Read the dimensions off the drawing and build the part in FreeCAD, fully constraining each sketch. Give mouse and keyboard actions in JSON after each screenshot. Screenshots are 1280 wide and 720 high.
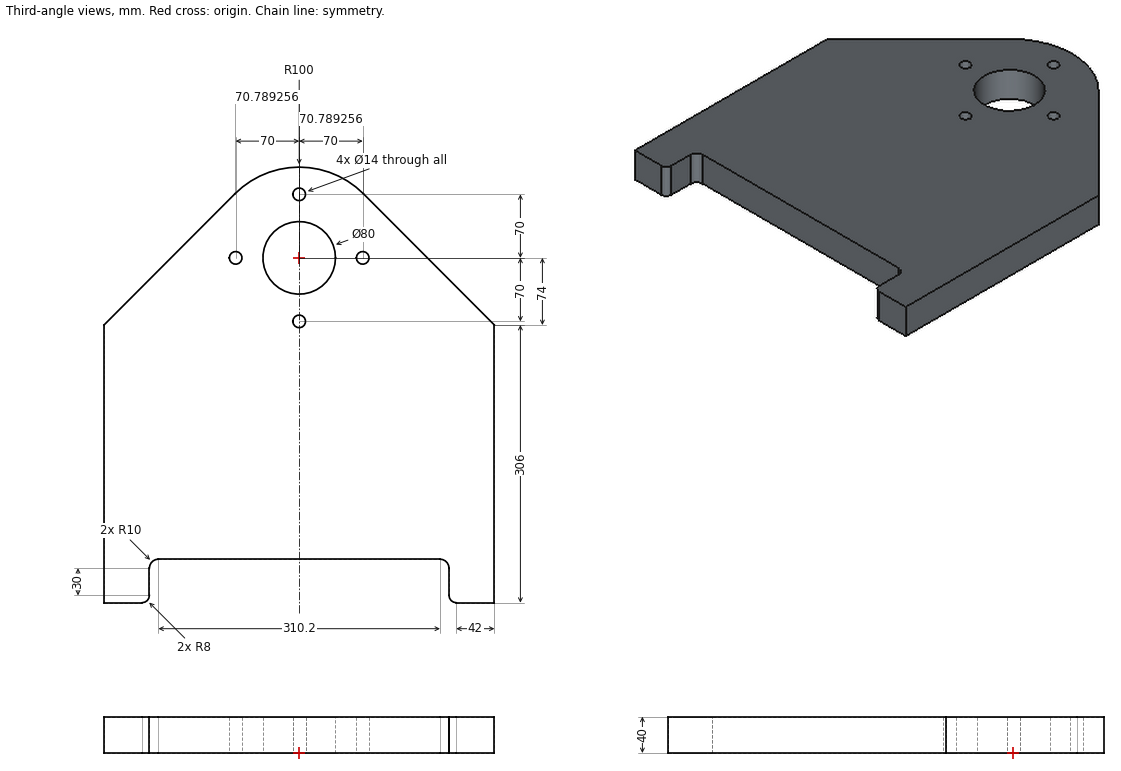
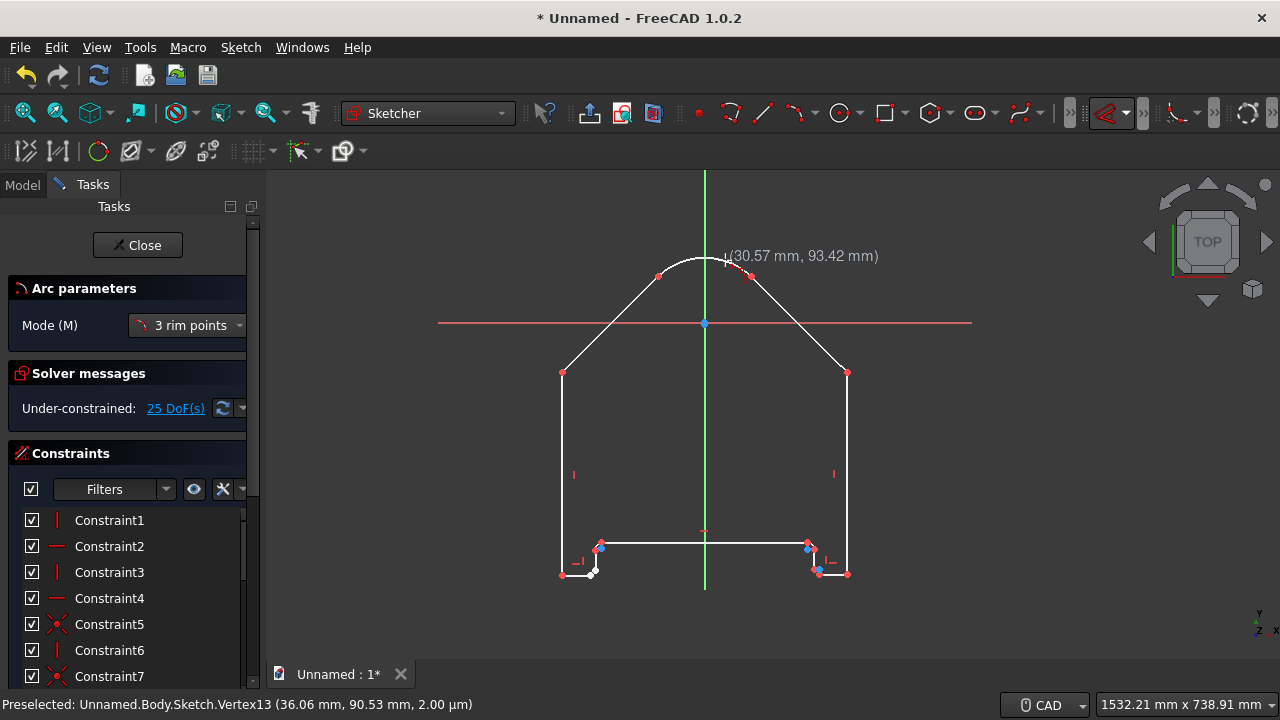
{"action": "scroll", "coordinate": [590, 574], "scroll_direction": "up", "scroll_amount": 4}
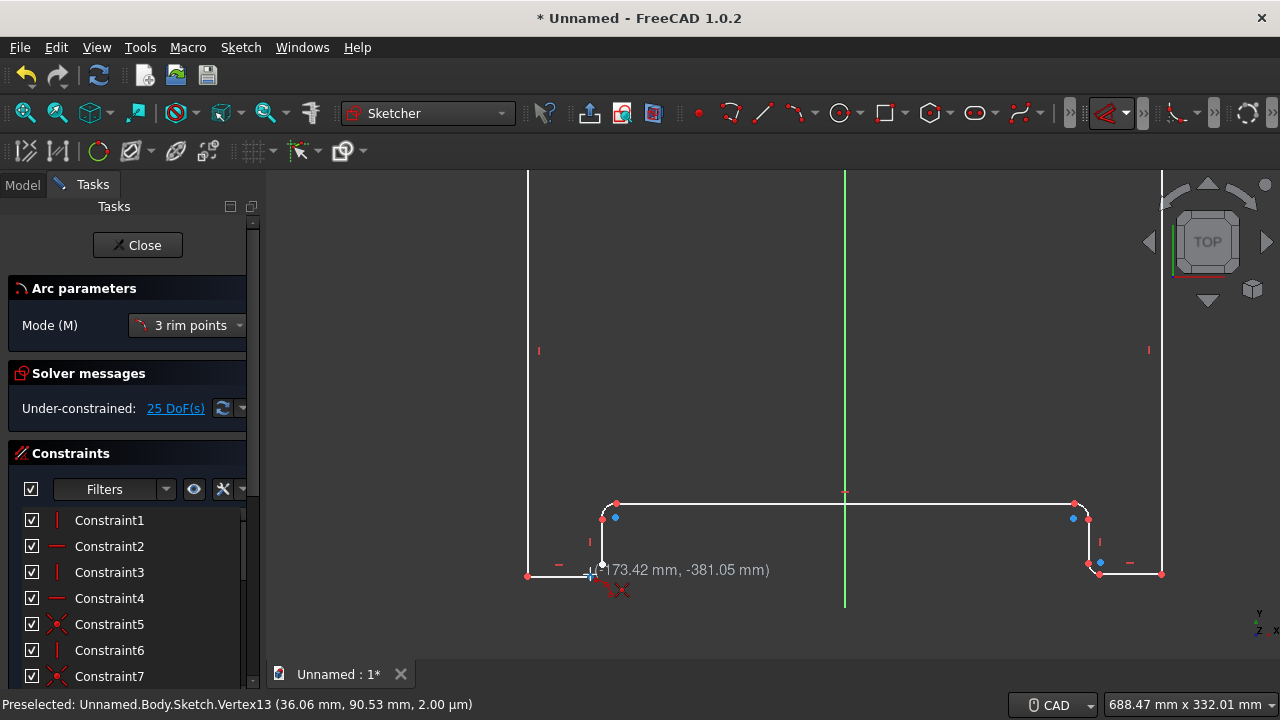
{"action": "left_click", "coordinate": [590, 577]}
{"action": "left_click", "coordinate": [602, 564]}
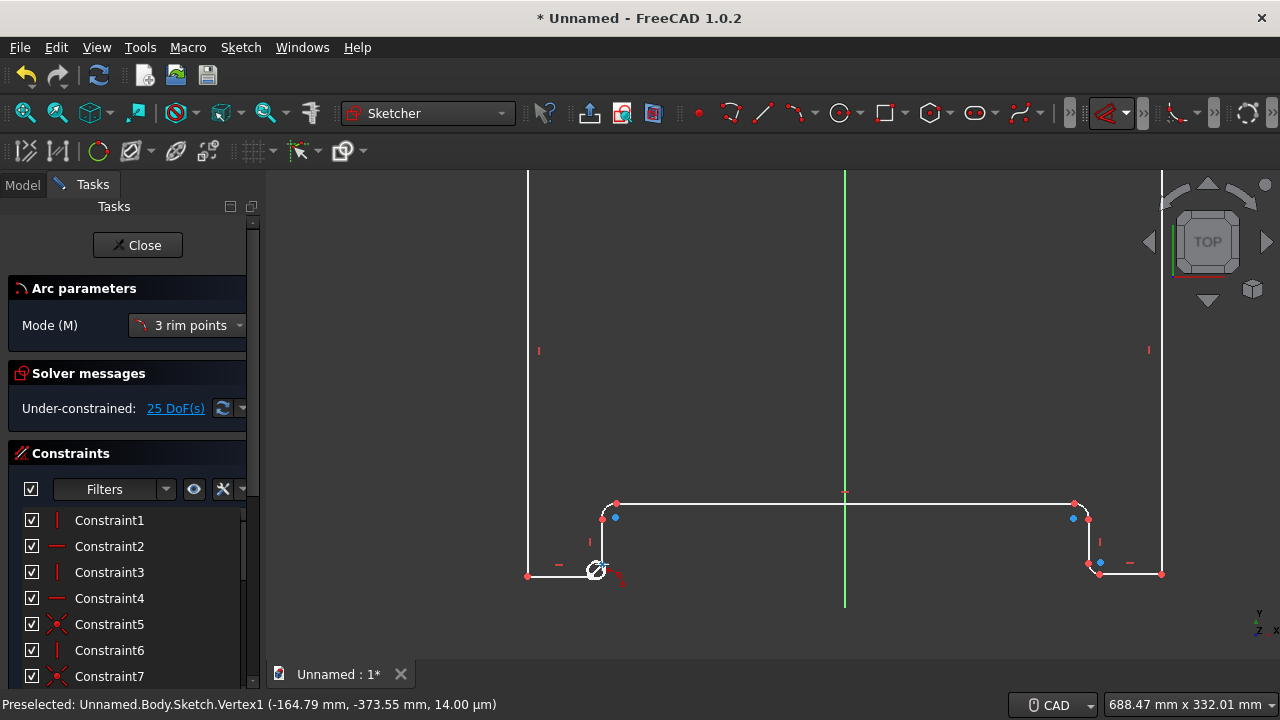
{"action": "scroll", "coordinate": [598, 570], "scroll_direction": "up", "scroll_amount": 8}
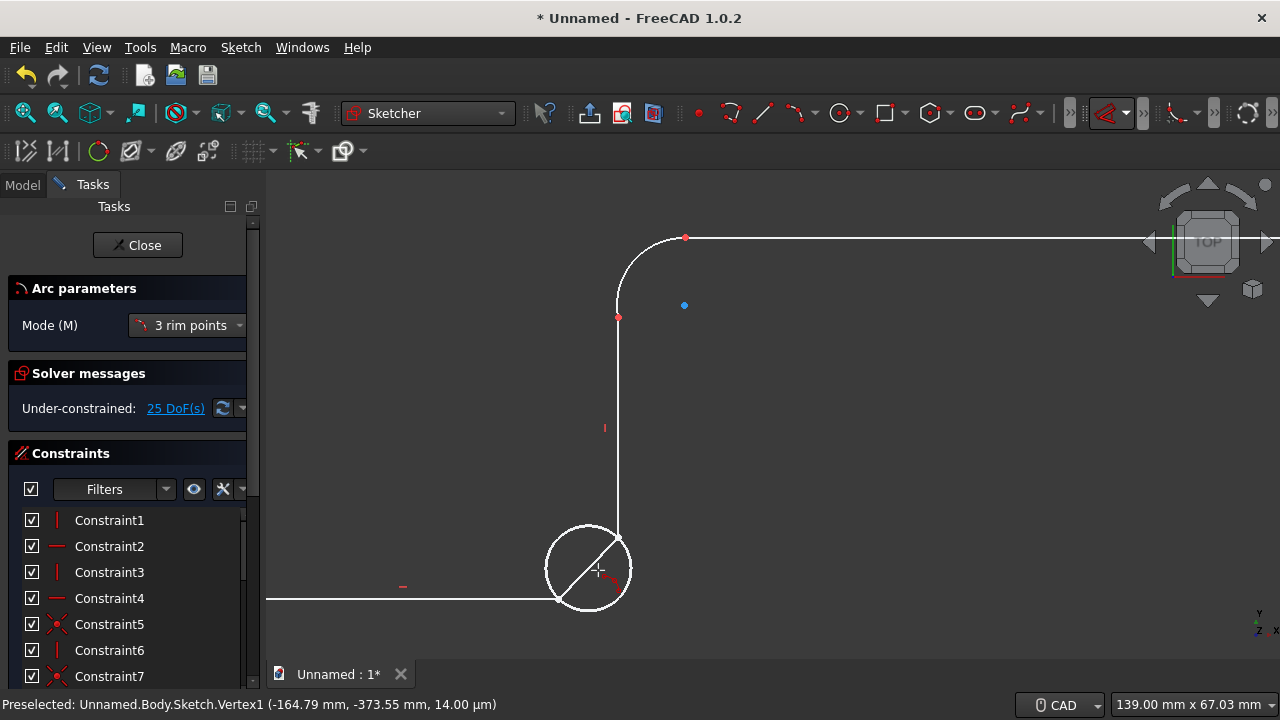
{"action": "left_click", "coordinate": [599, 568]}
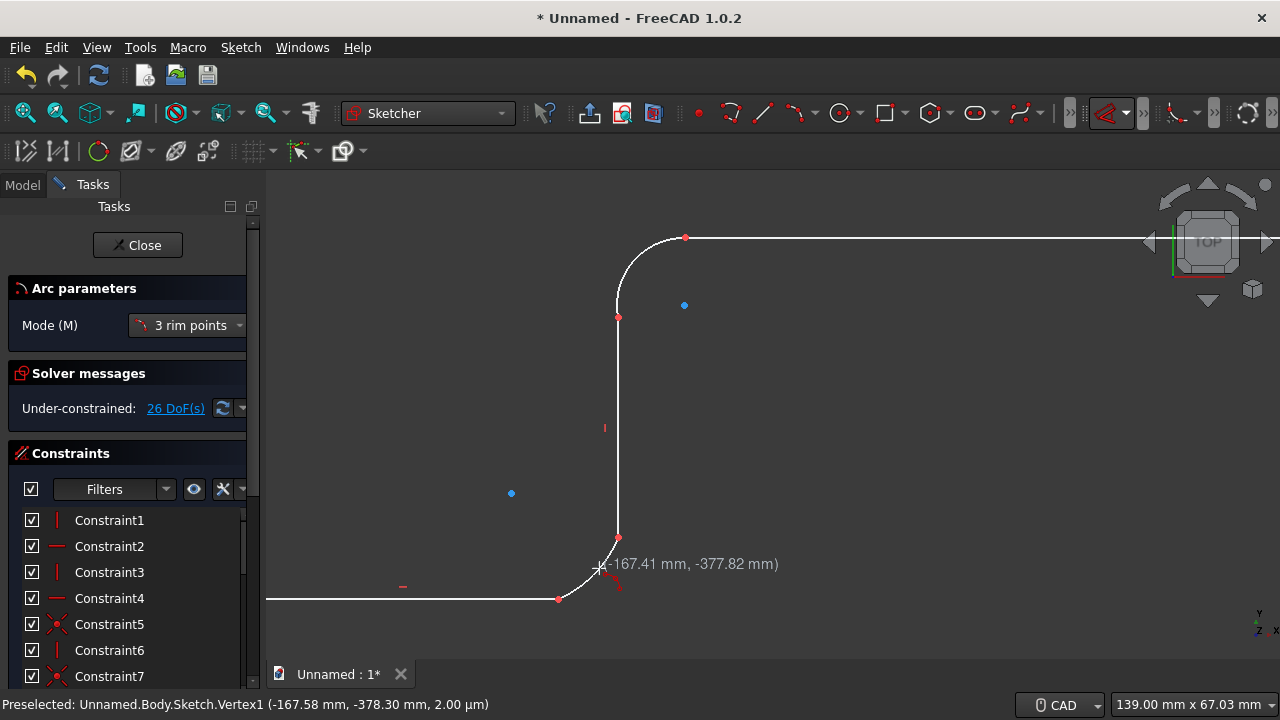
{"action": "key", "text": "g c"}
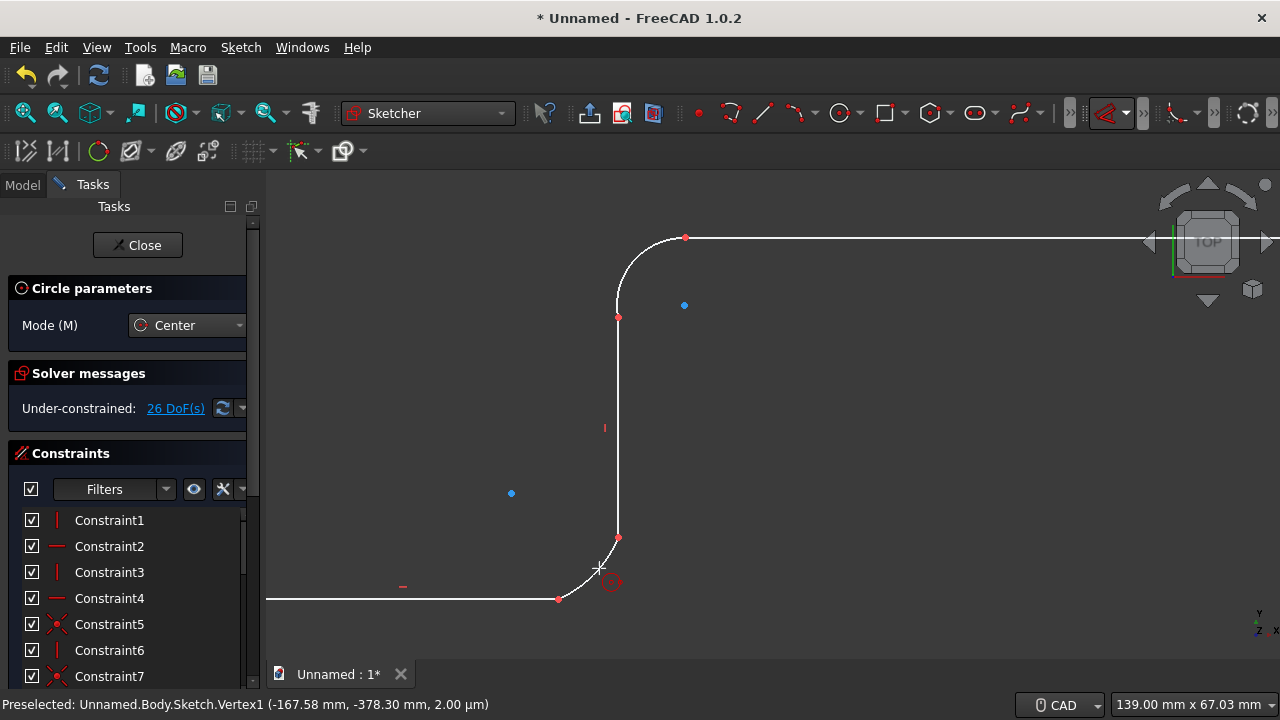
{"action": "scroll", "coordinate": [593, 572], "scroll_direction": "down", "scroll_amount": 12}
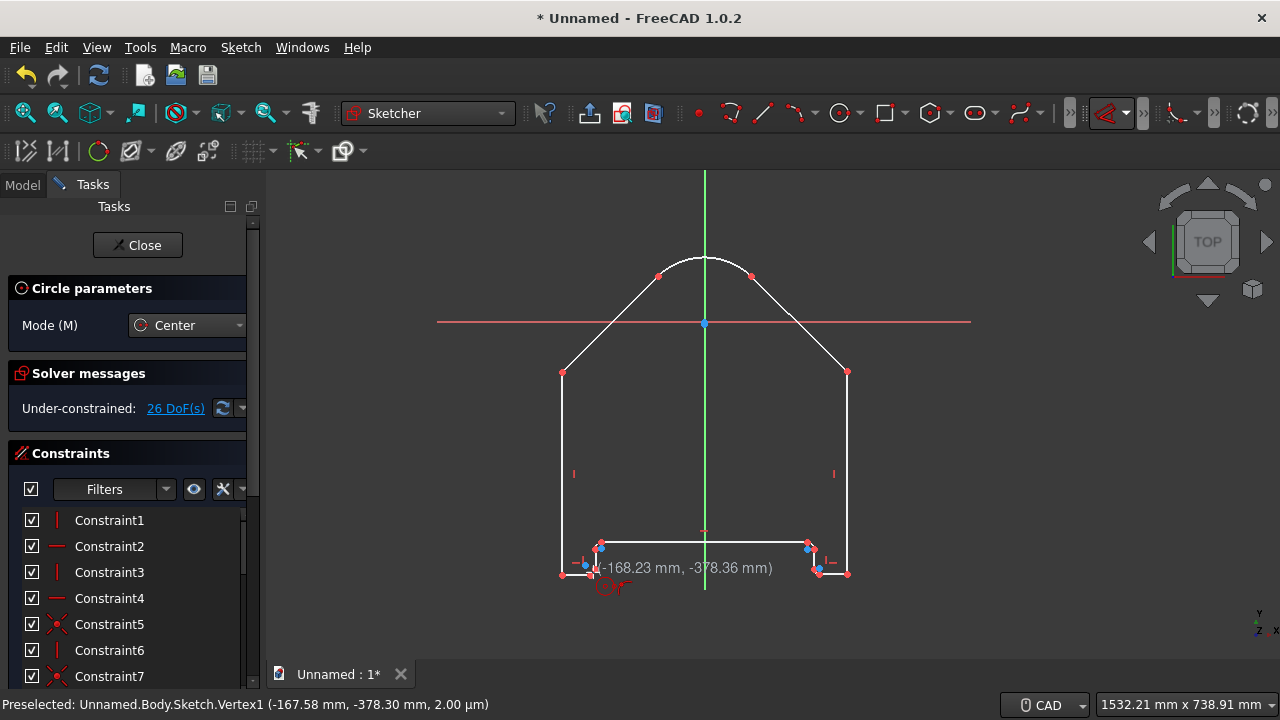
{"action": "left_click", "coordinate": [705, 322]}
{"action": "left_click", "coordinate": [723, 304]}
{"action": "key", "text": "Escape"}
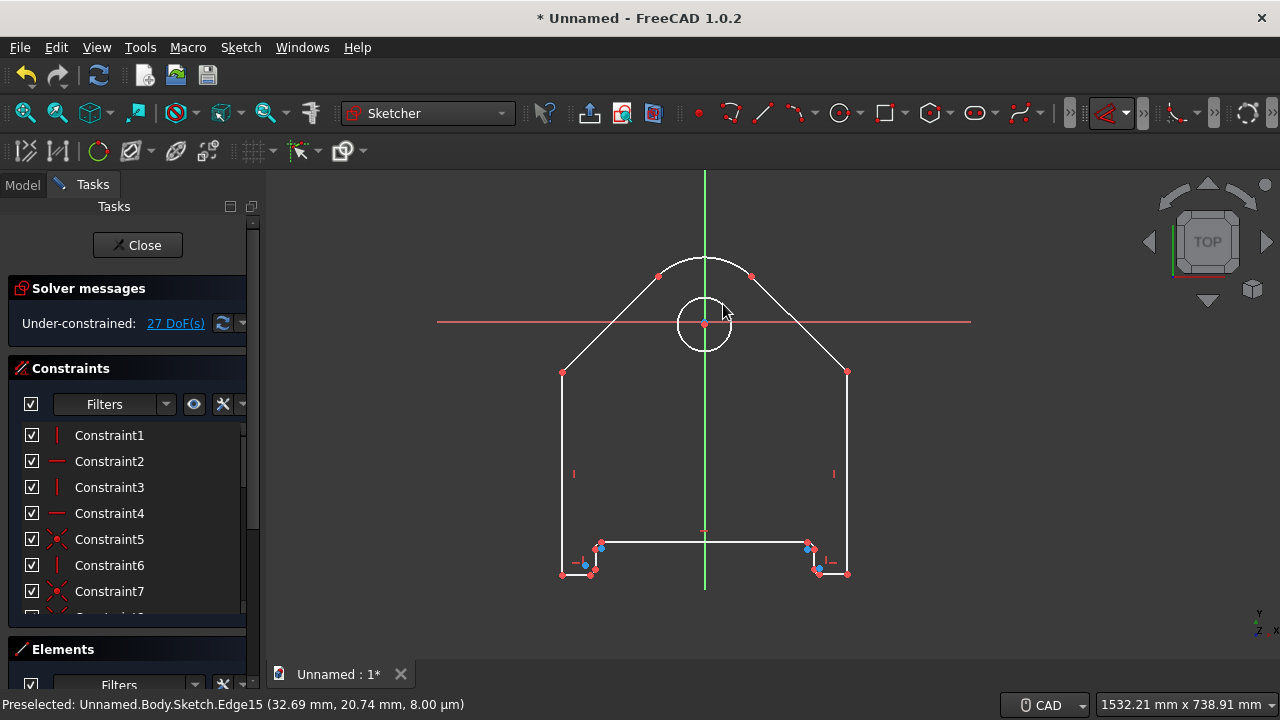
{"action": "scroll", "coordinate": [596, 560], "scroll_direction": "up", "scroll_amount": 2}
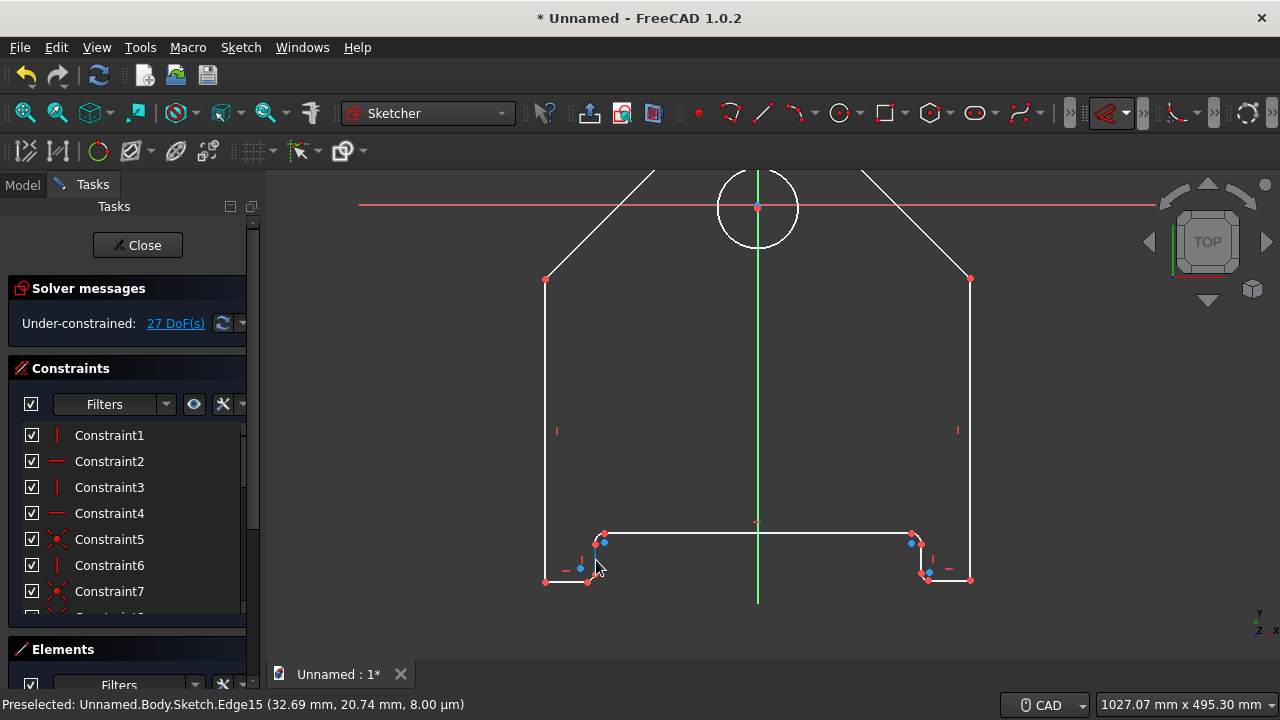
{"action": "left_click", "coordinate": [595, 559]}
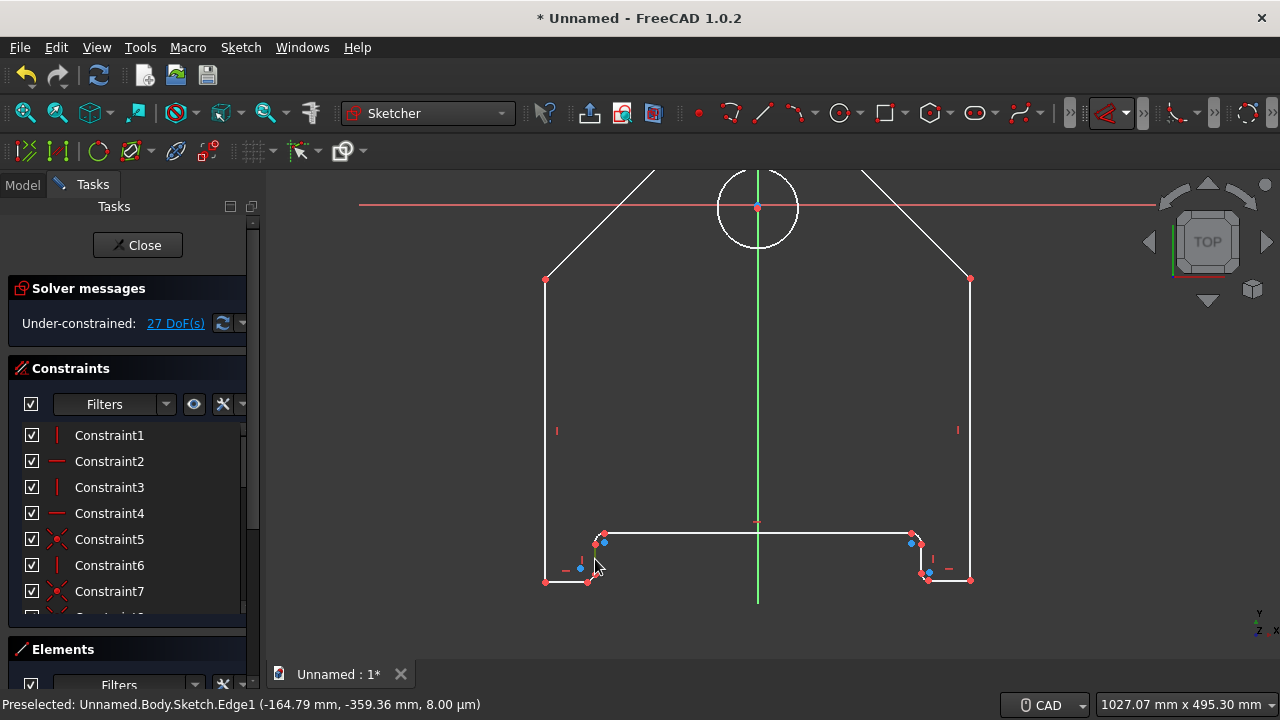
{"action": "scroll", "coordinate": [597, 537], "scroll_direction": "up", "scroll_amount": 3}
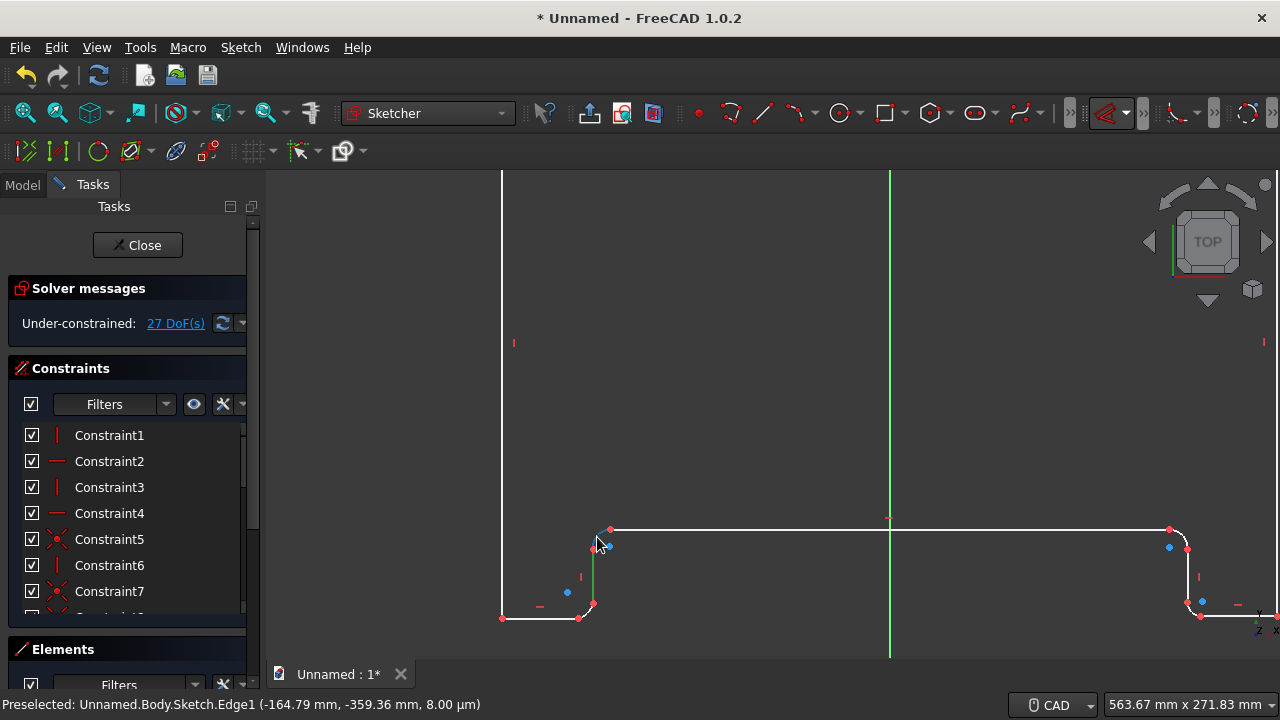
{"action": "left_click", "coordinate": [597, 536]}